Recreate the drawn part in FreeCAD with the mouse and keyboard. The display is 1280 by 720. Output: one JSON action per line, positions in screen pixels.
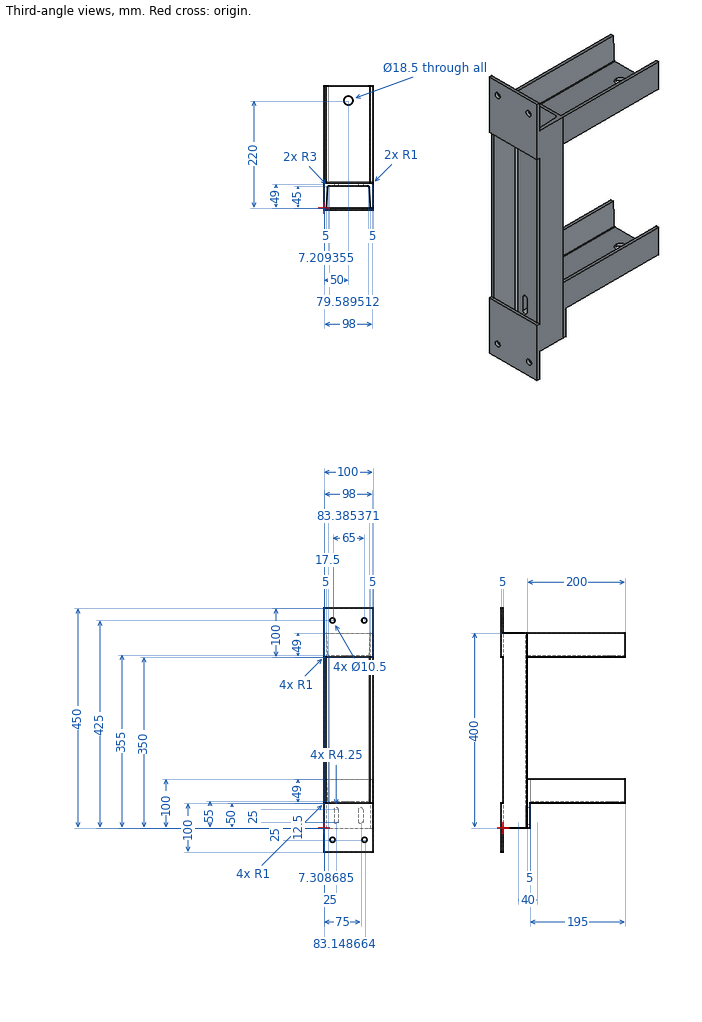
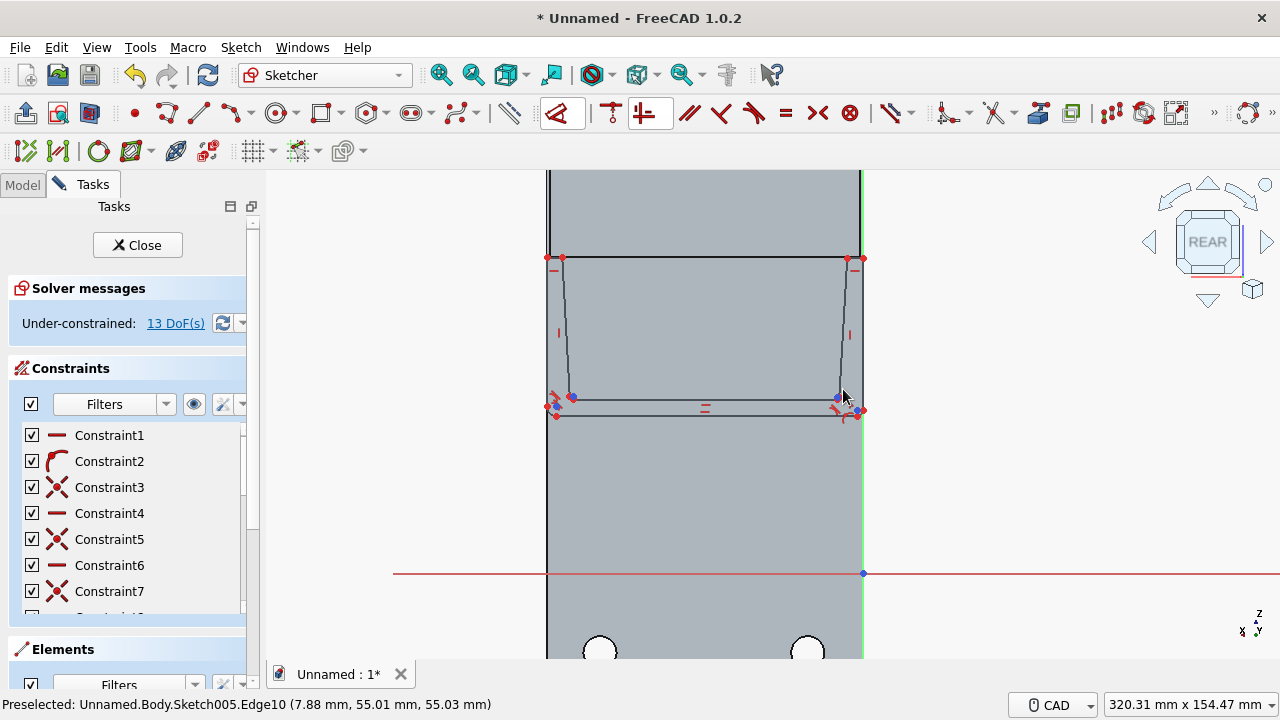
{"action": "scroll", "coordinate": [570, 398], "scroll_direction": "up", "scroll_amount": 11}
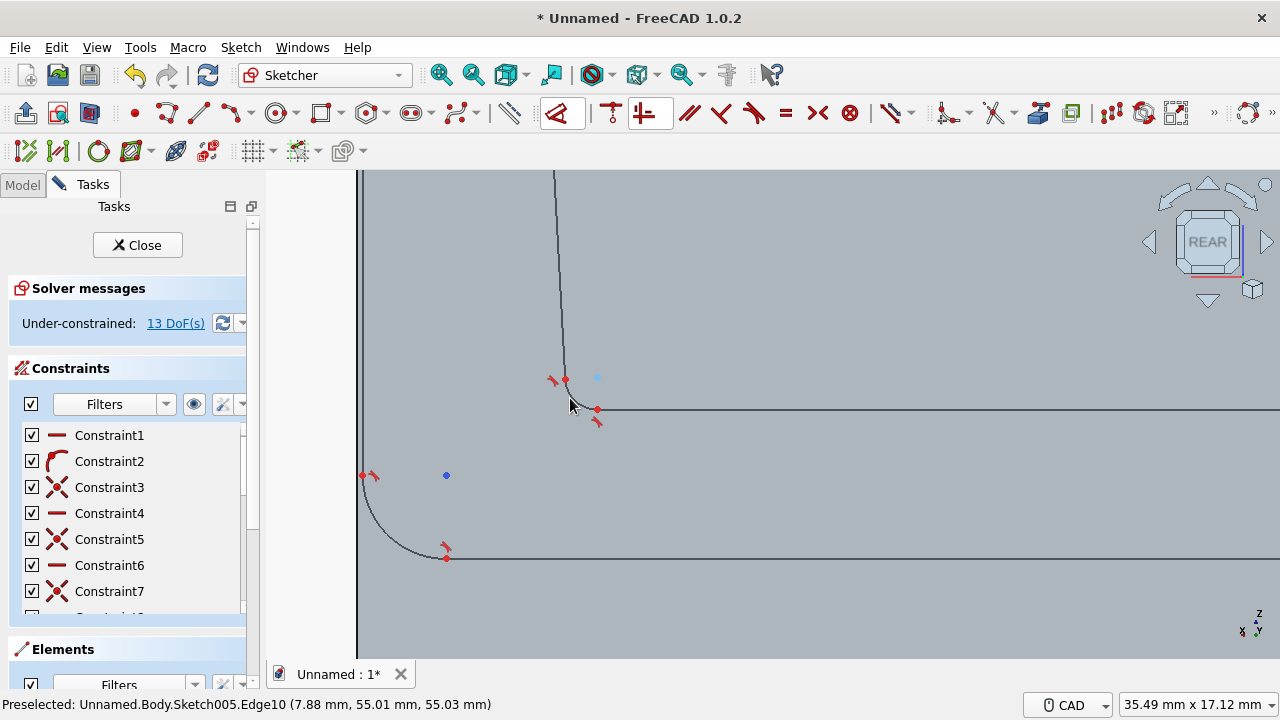
{"action": "left_click", "coordinate": [569, 393]}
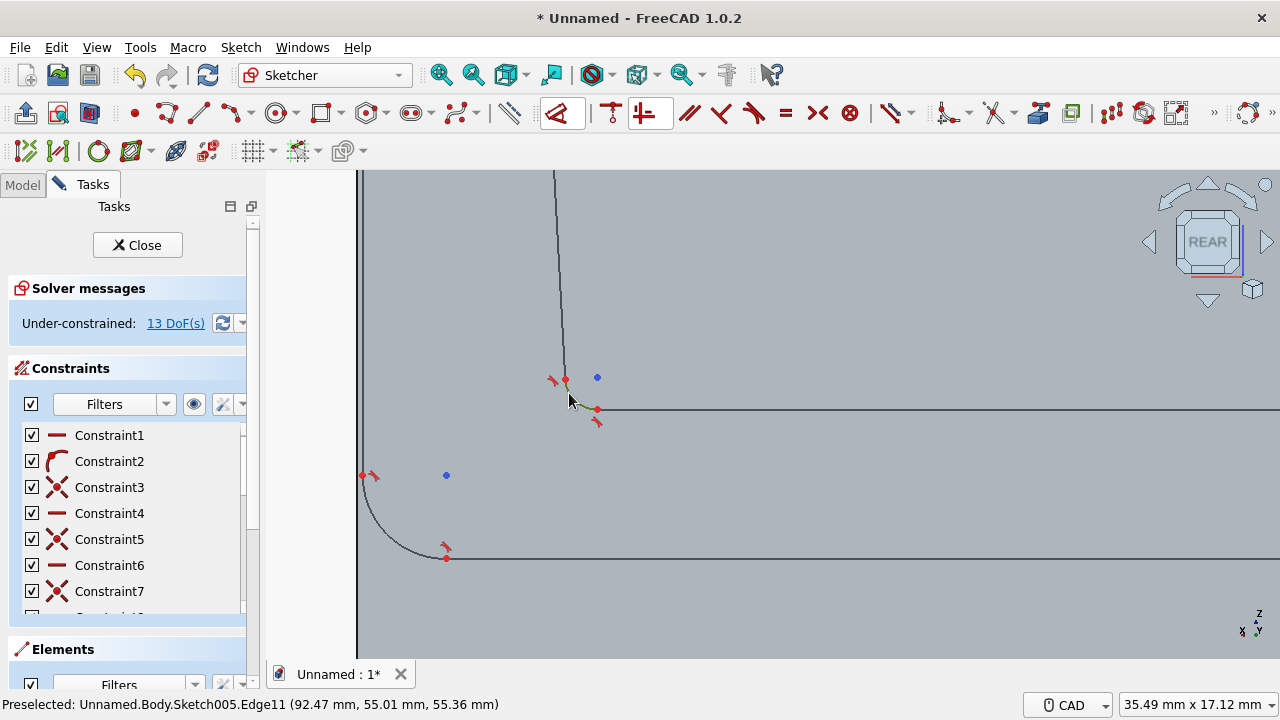
{"action": "left_click", "coordinate": [372, 513]}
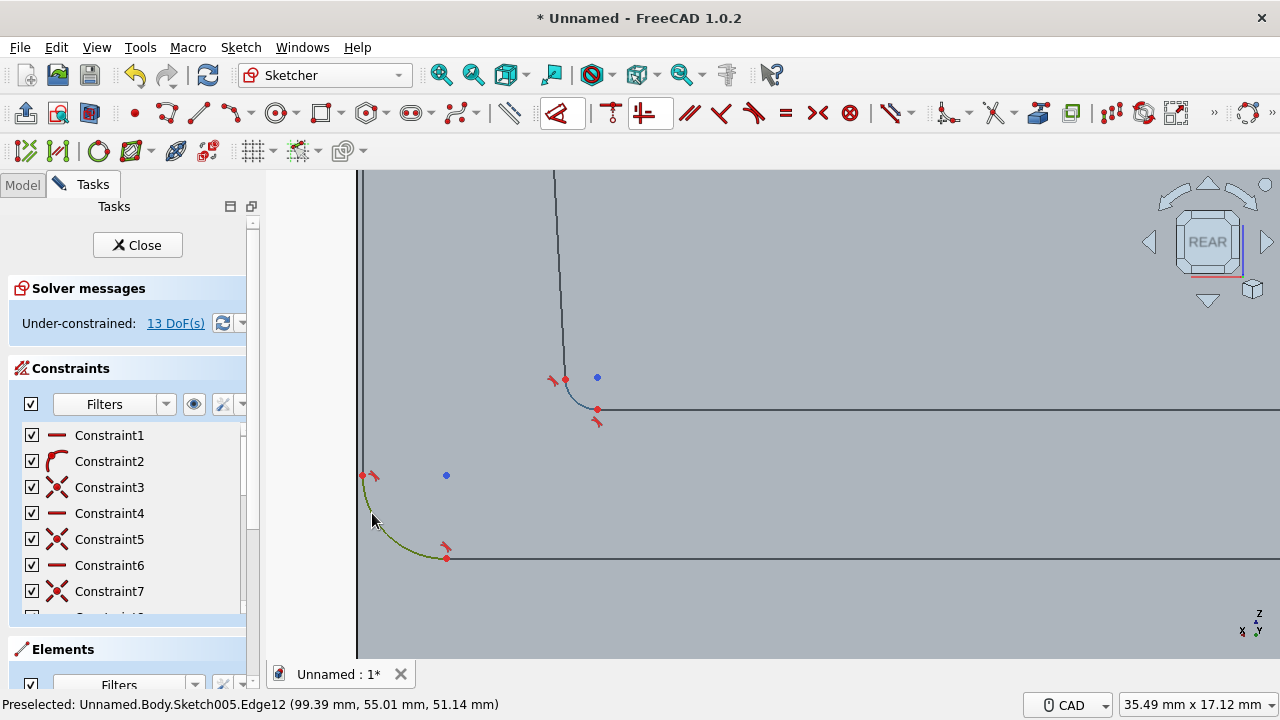
{"action": "left_click", "coordinate": [786, 114]}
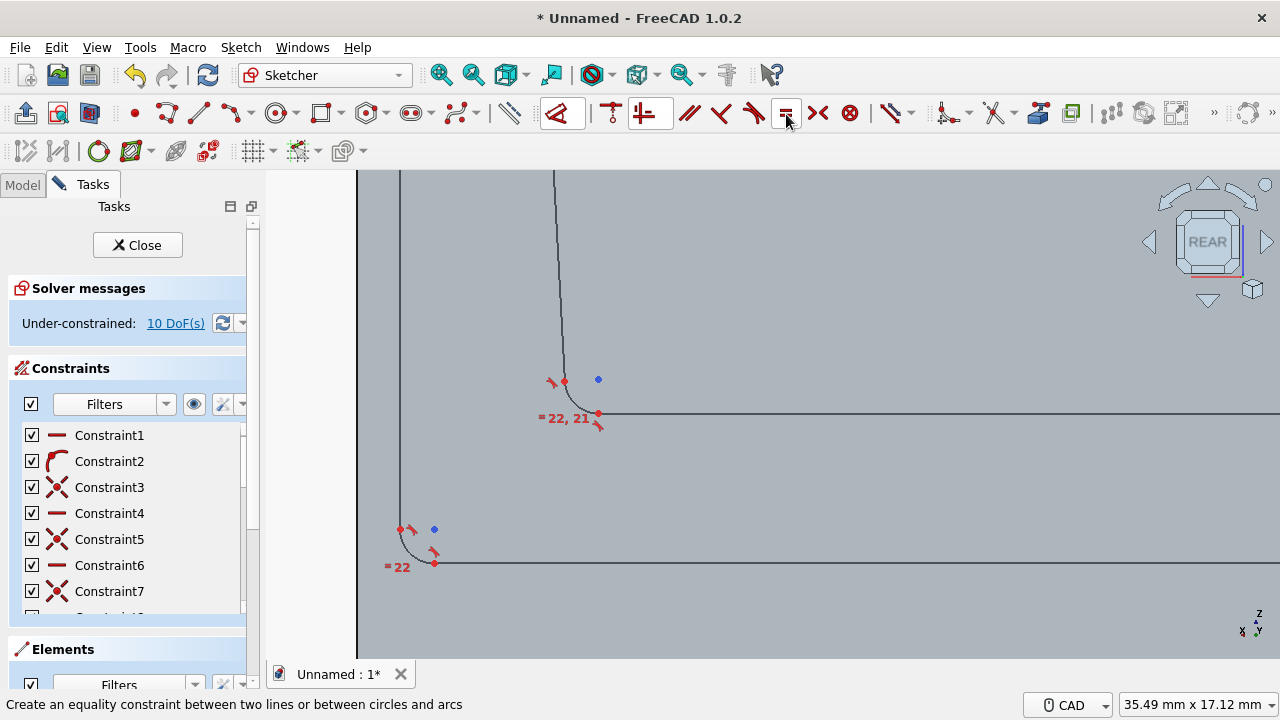
{"action": "scroll", "coordinate": [570, 398], "scroll_direction": "down", "scroll_amount": 11}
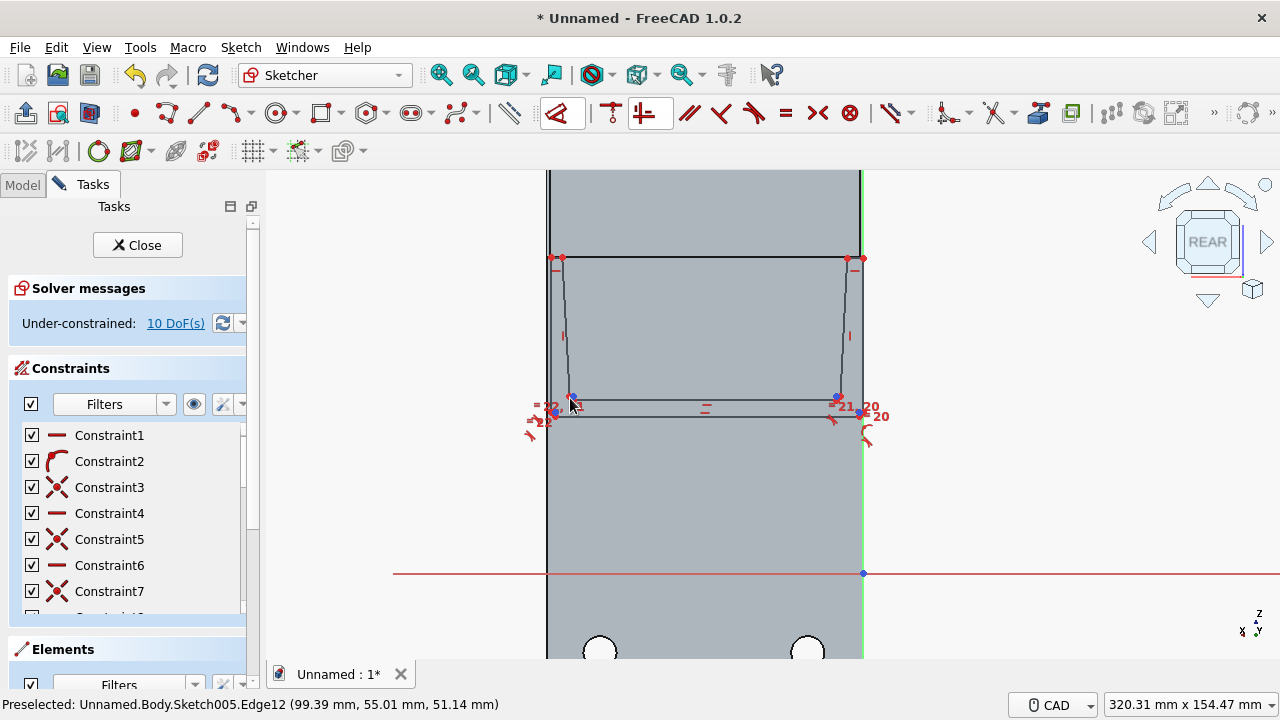
{"action": "scroll", "coordinate": [861, 416], "scroll_direction": "up", "scroll_amount": 13}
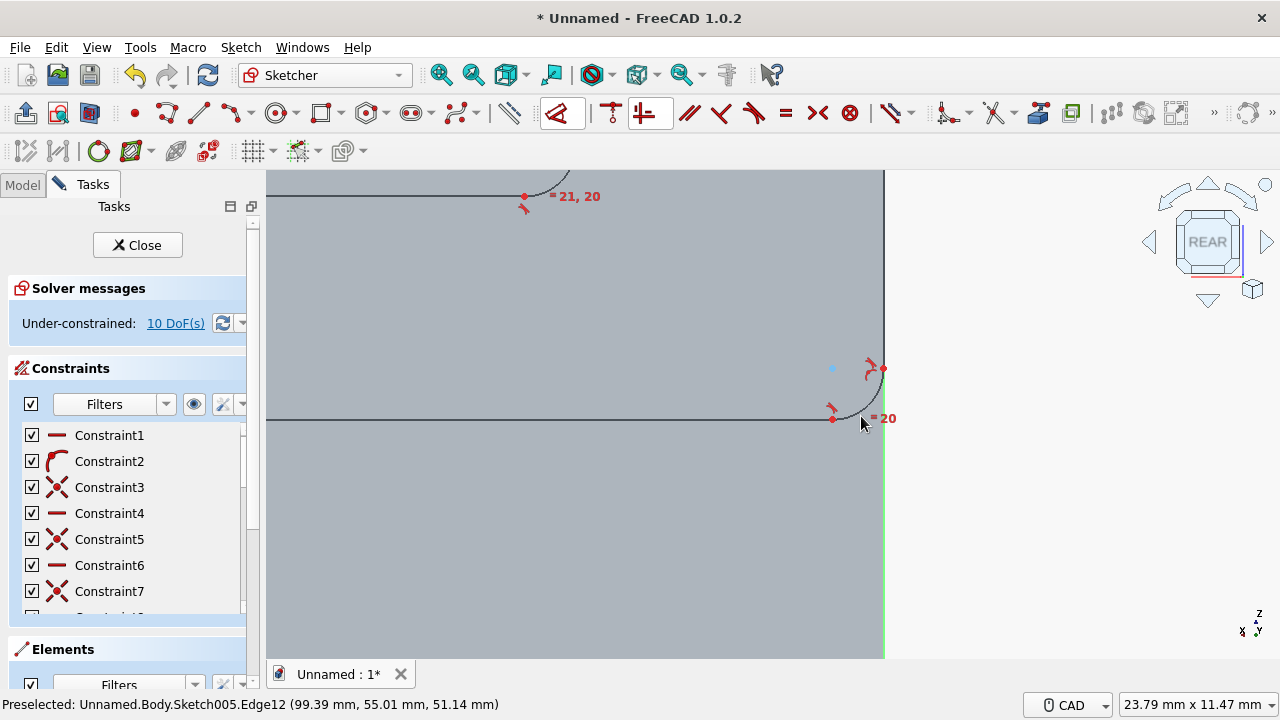
{"action": "left_click", "coordinate": [856, 414]}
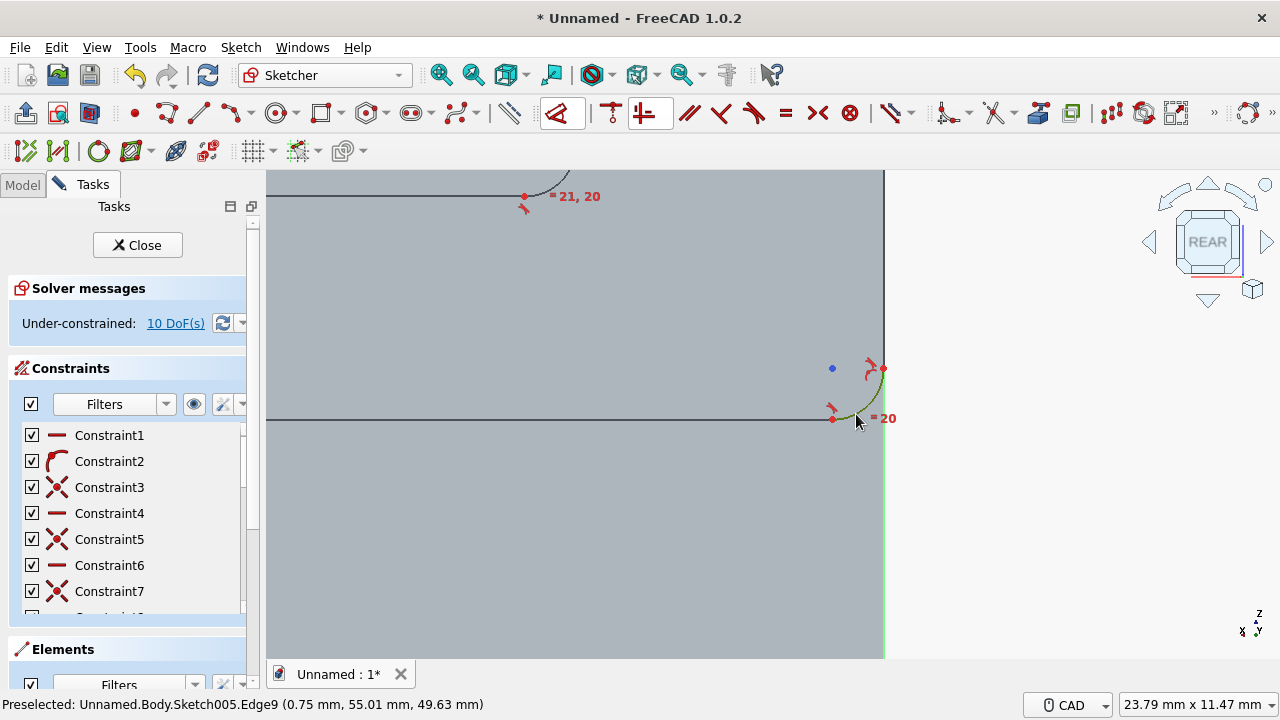
{"action": "key", "text": "k r"}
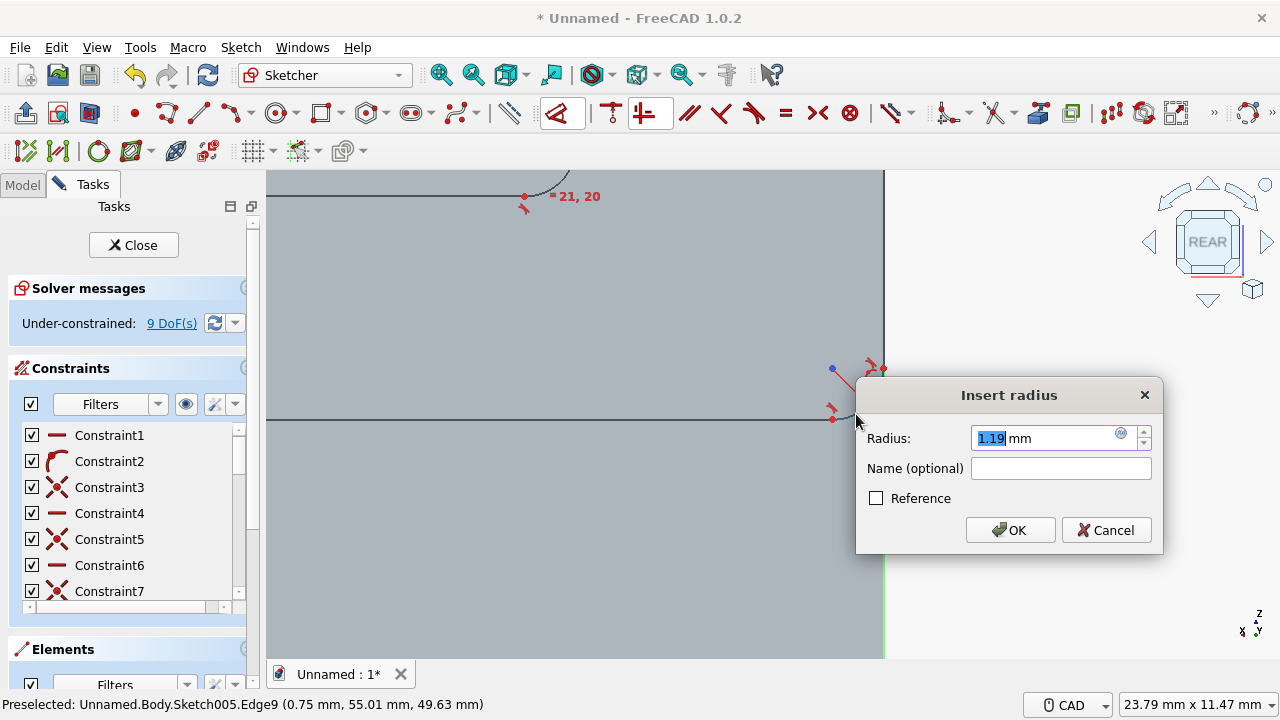
{"action": "type", "text": "1"}
{"action": "key", "text": "Return"}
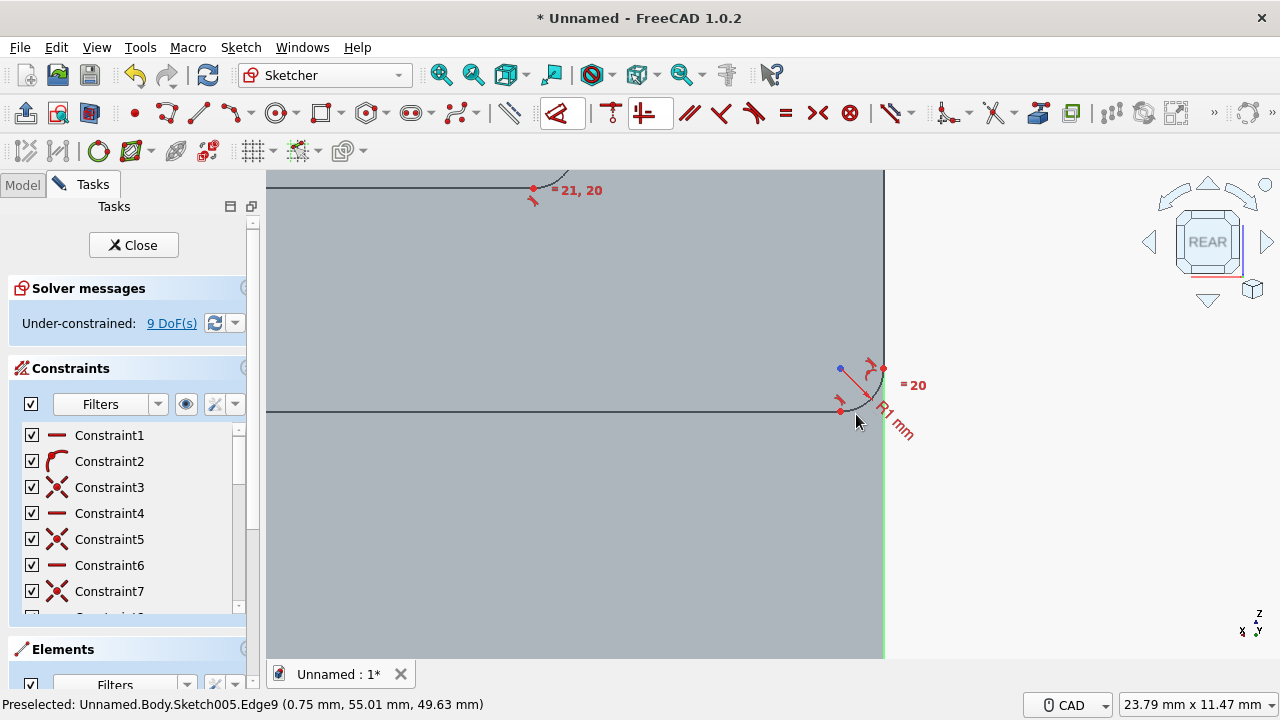
{"action": "scroll", "coordinate": [861, 416], "scroll_direction": "down", "scroll_amount": 13}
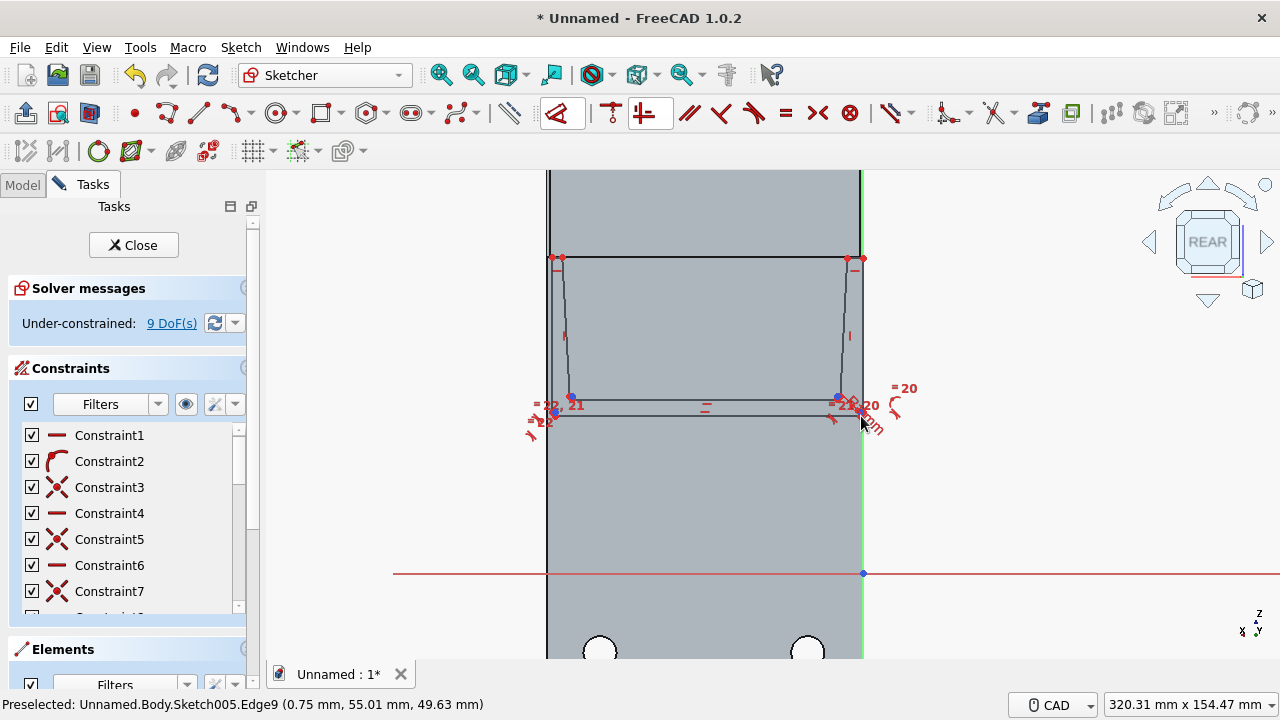
{"action": "scroll", "coordinate": [858, 258], "scroll_direction": "up", "scroll_amount": 6}